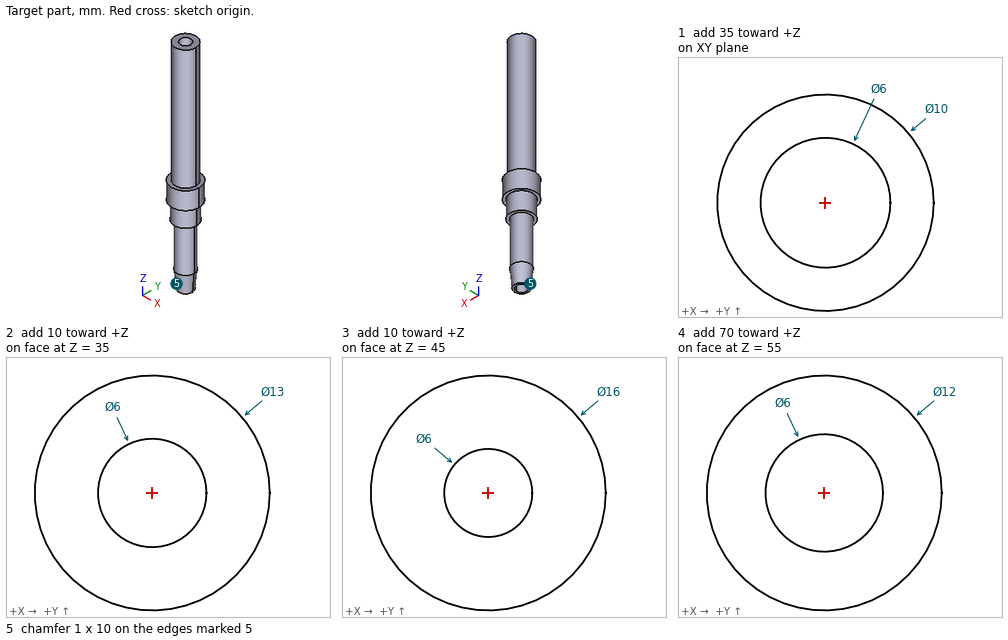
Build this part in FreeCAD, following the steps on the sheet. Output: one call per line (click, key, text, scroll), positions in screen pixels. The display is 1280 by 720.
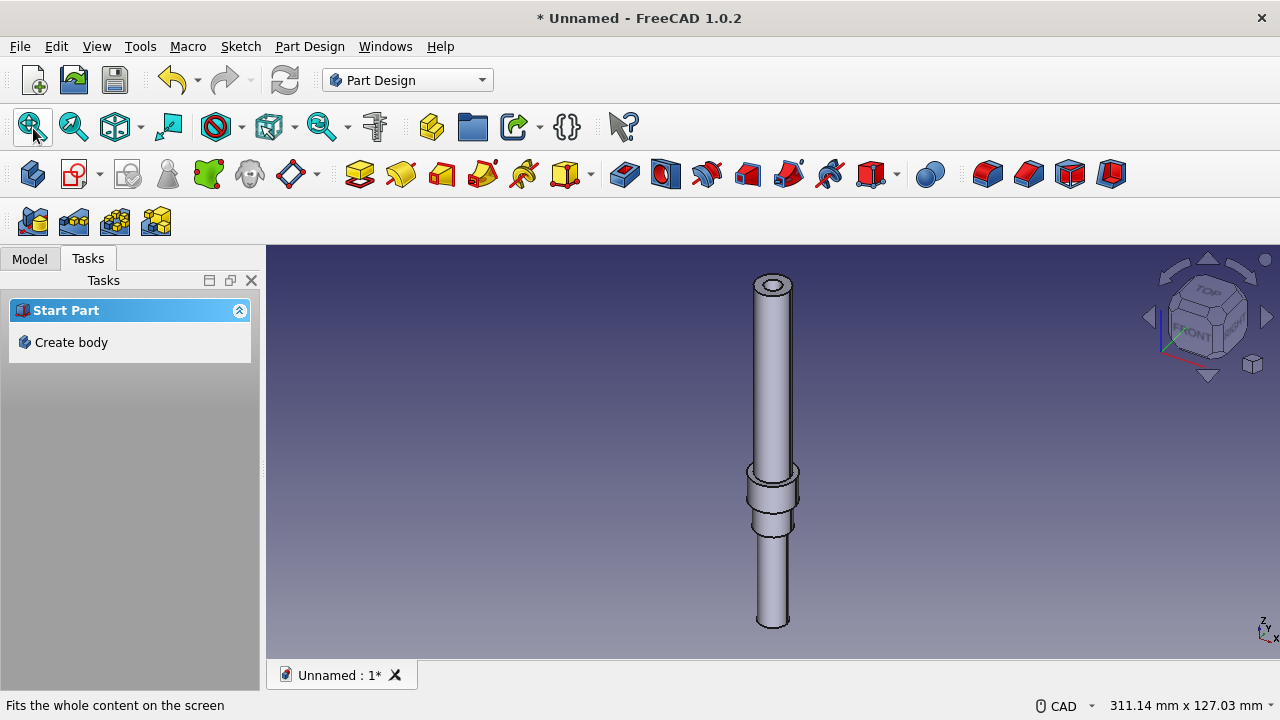
key(0)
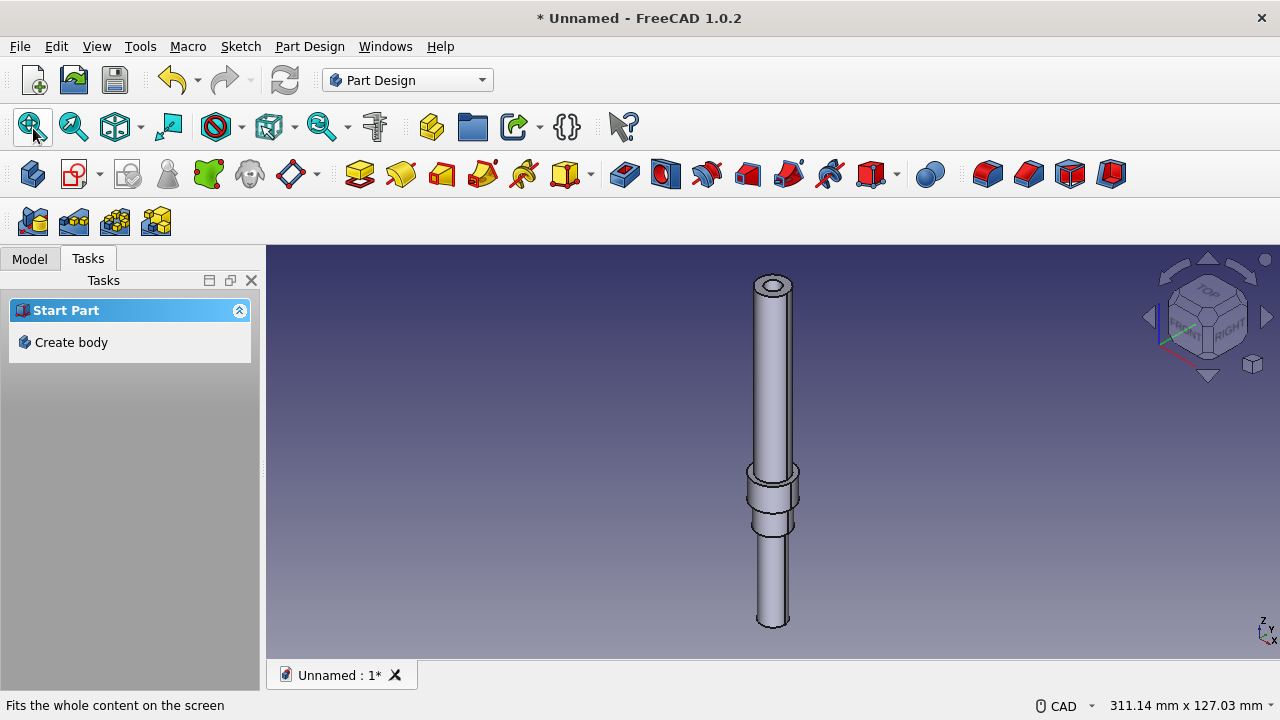
click(758, 622)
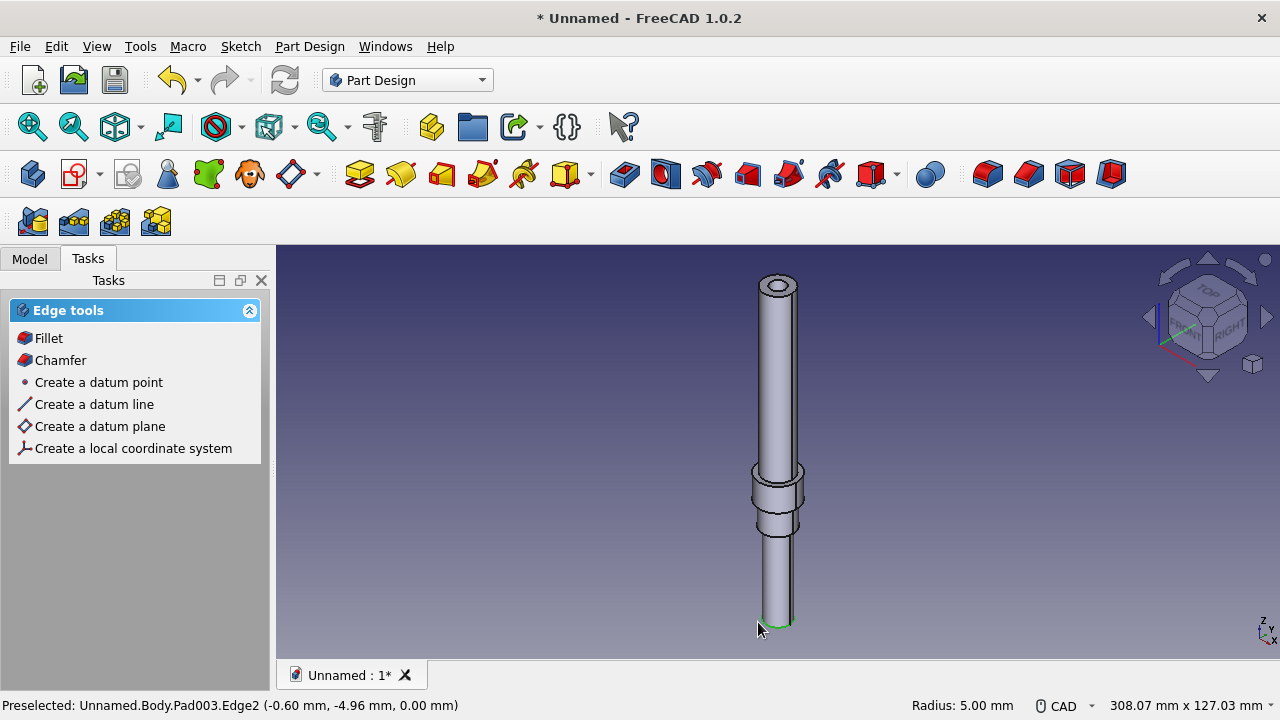
click(1029, 174)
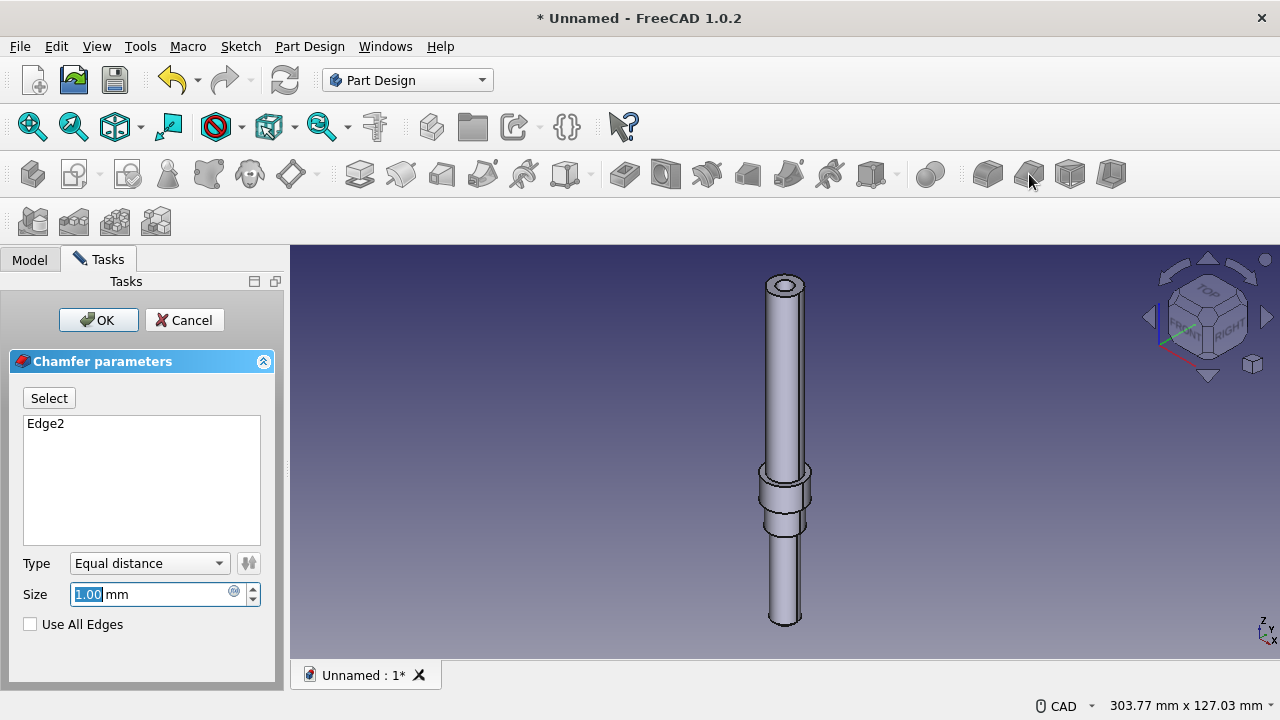
text(1)
key(Tab)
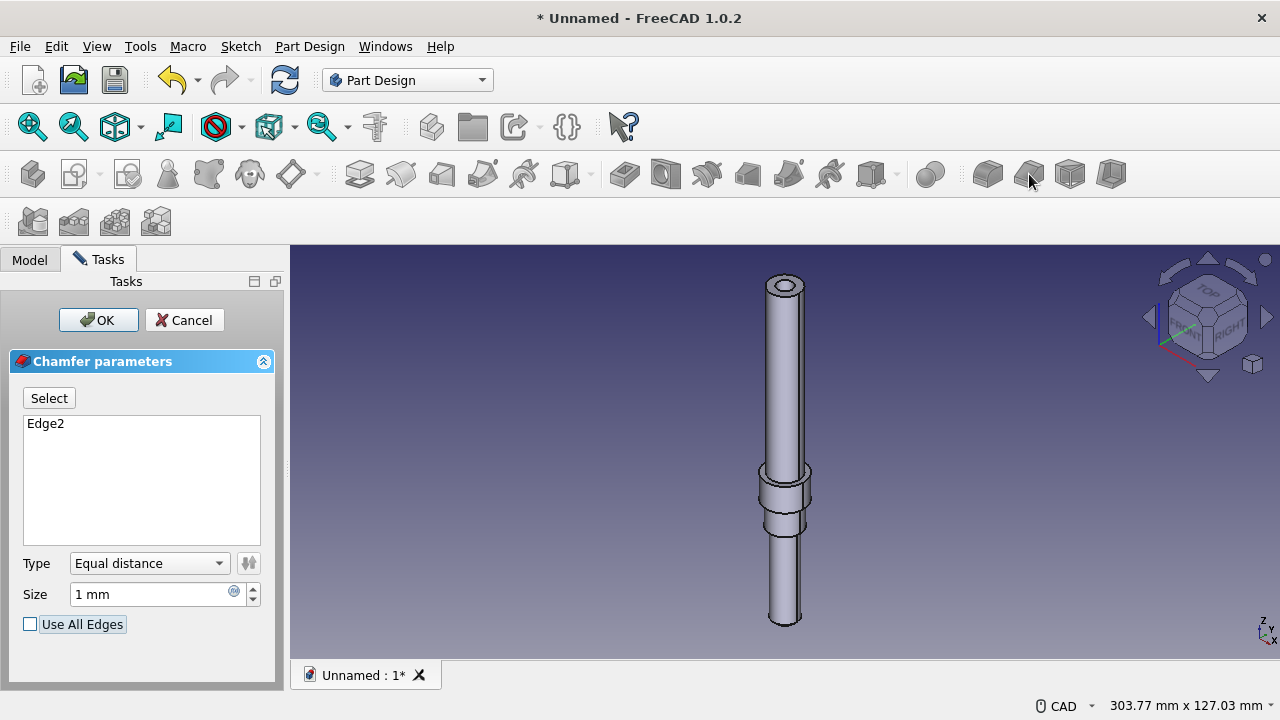
click(150, 564)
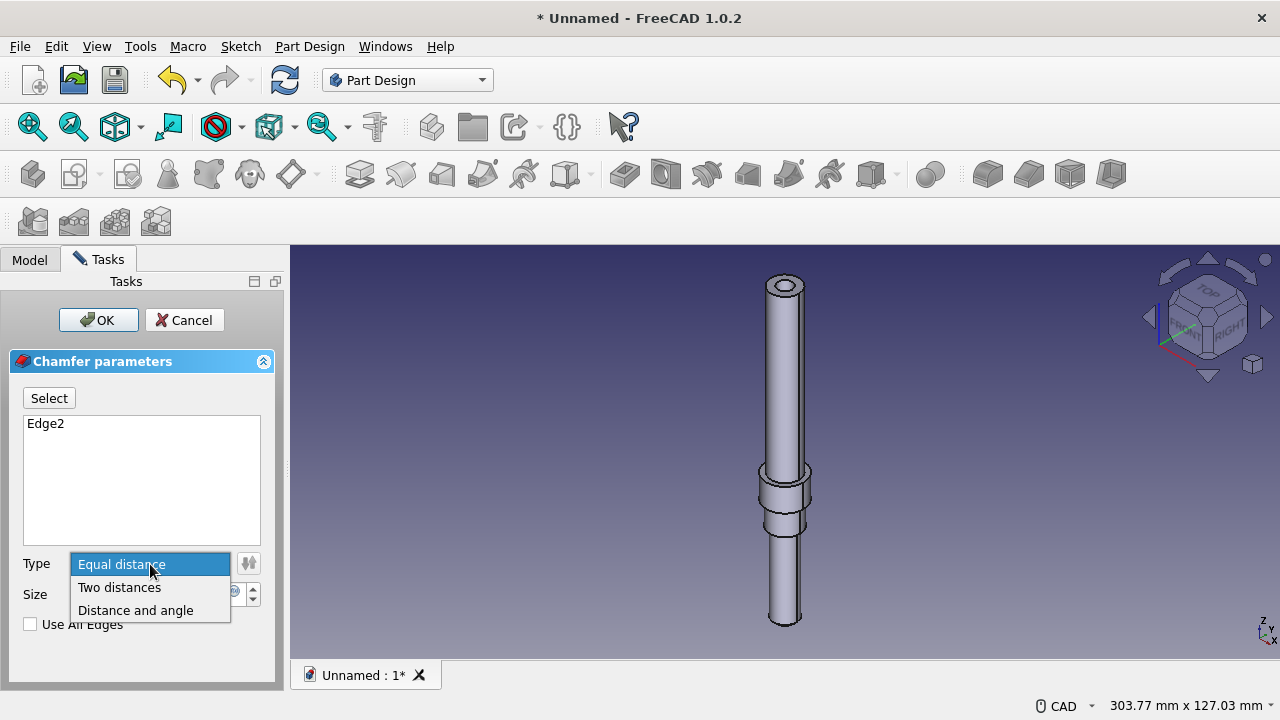
click(148, 588)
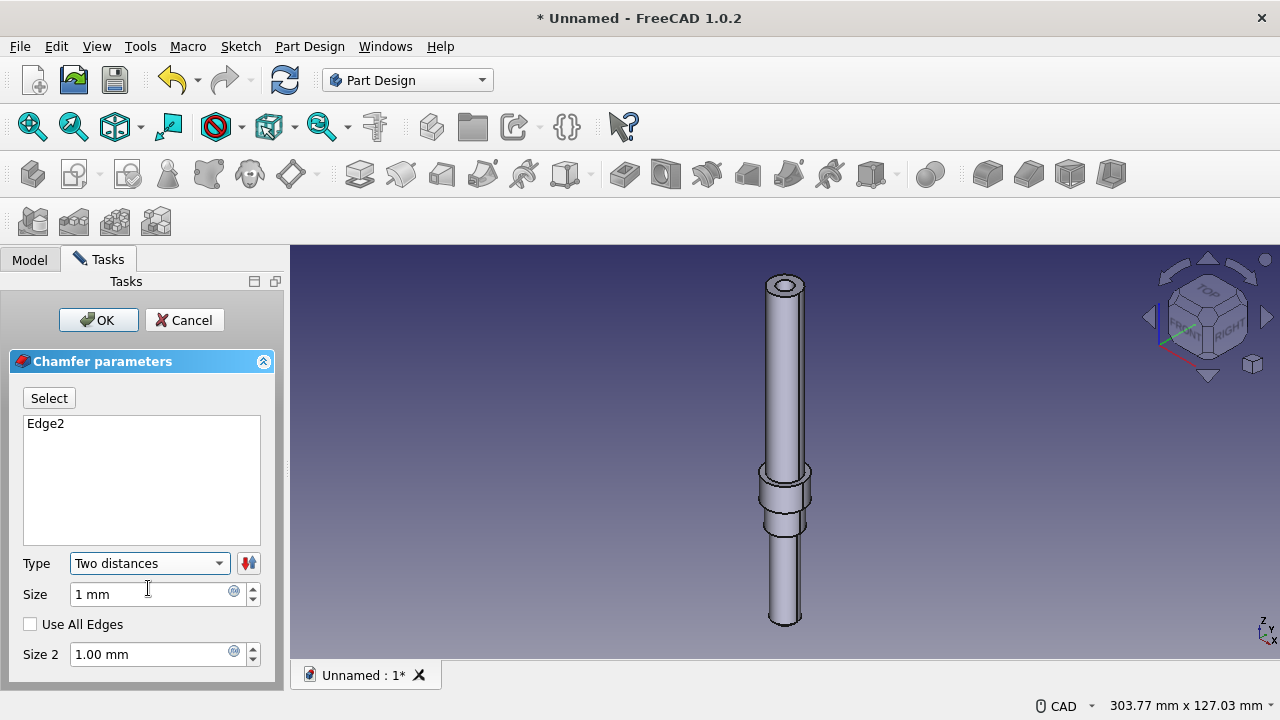
triple_click(158, 654)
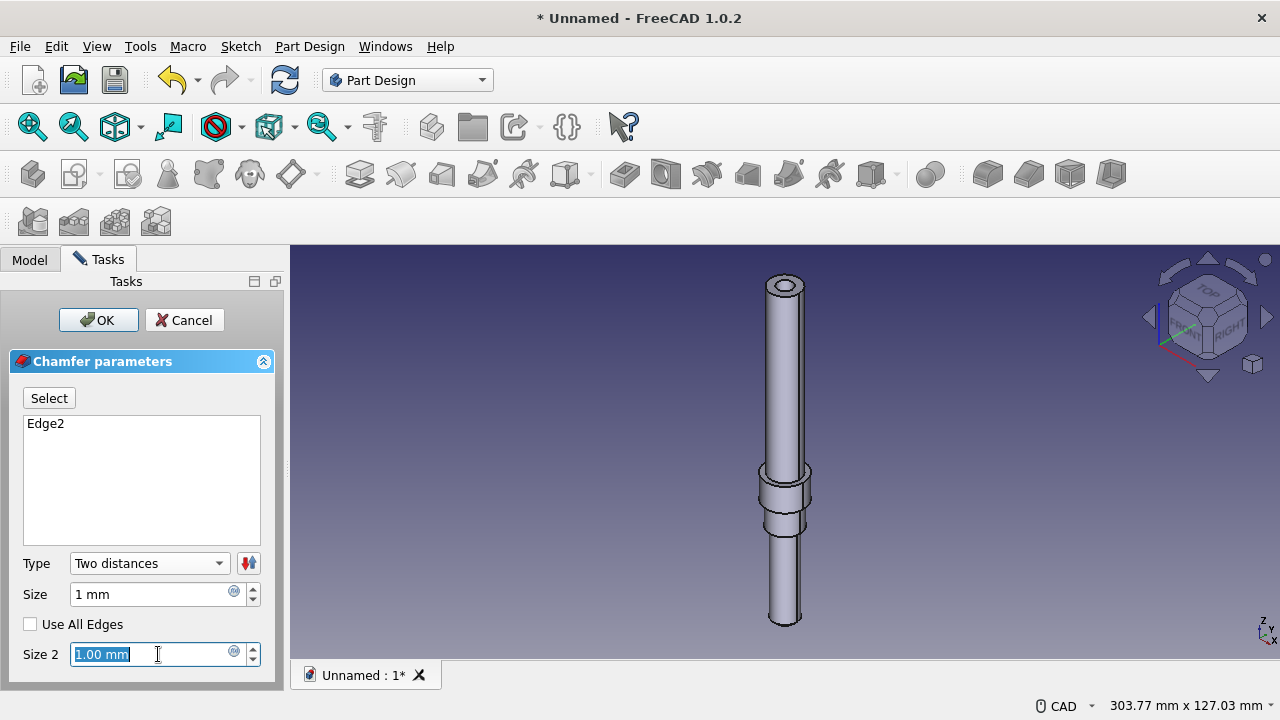
text(10)
key(Tab)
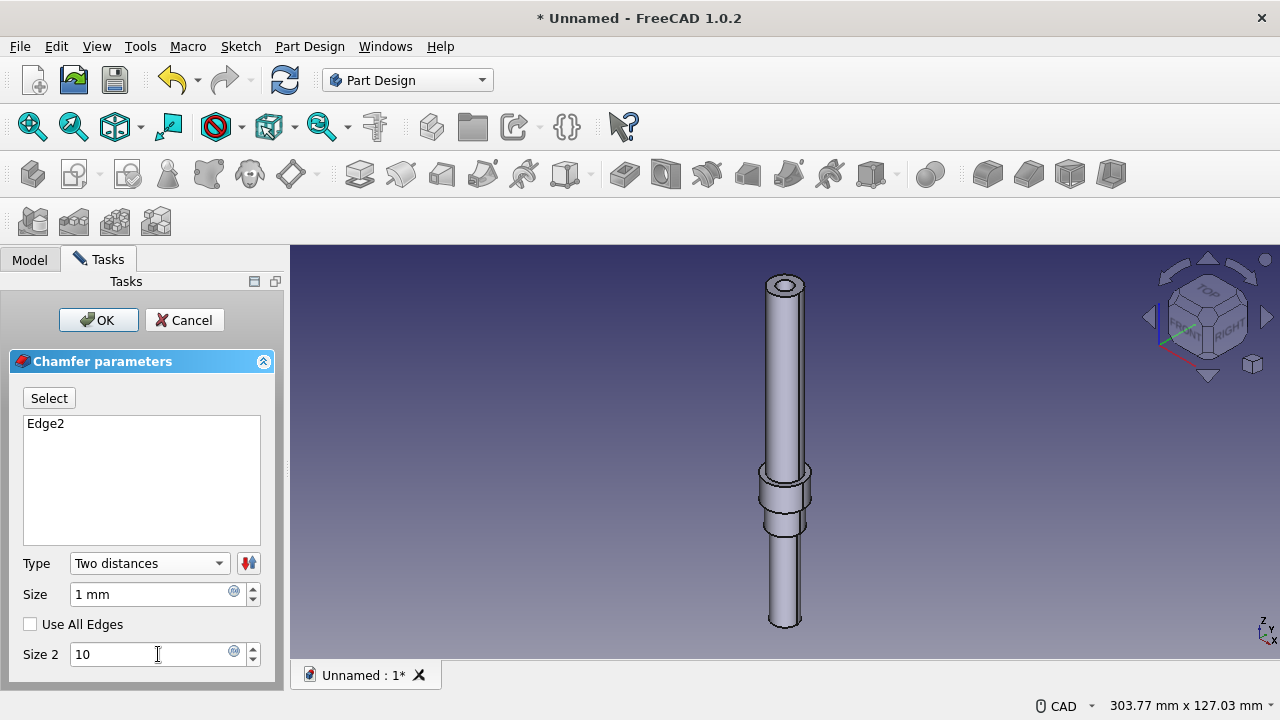
click(249, 564)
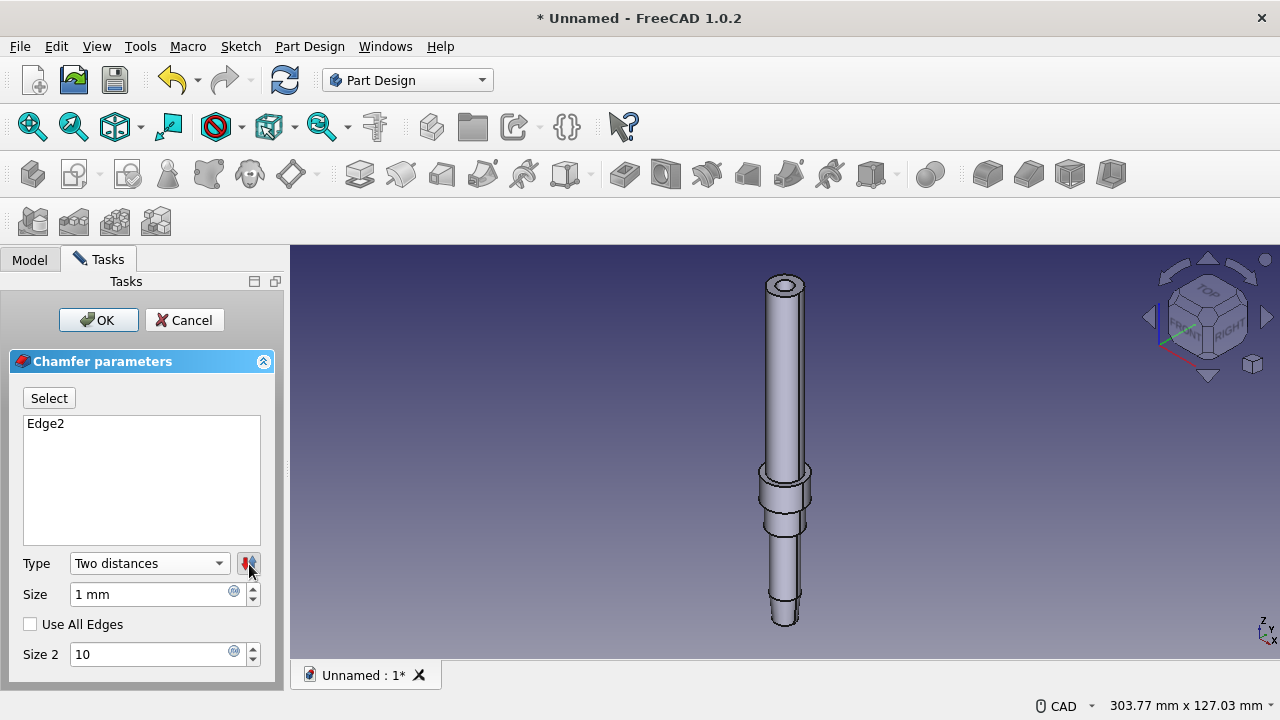
click(99, 320)